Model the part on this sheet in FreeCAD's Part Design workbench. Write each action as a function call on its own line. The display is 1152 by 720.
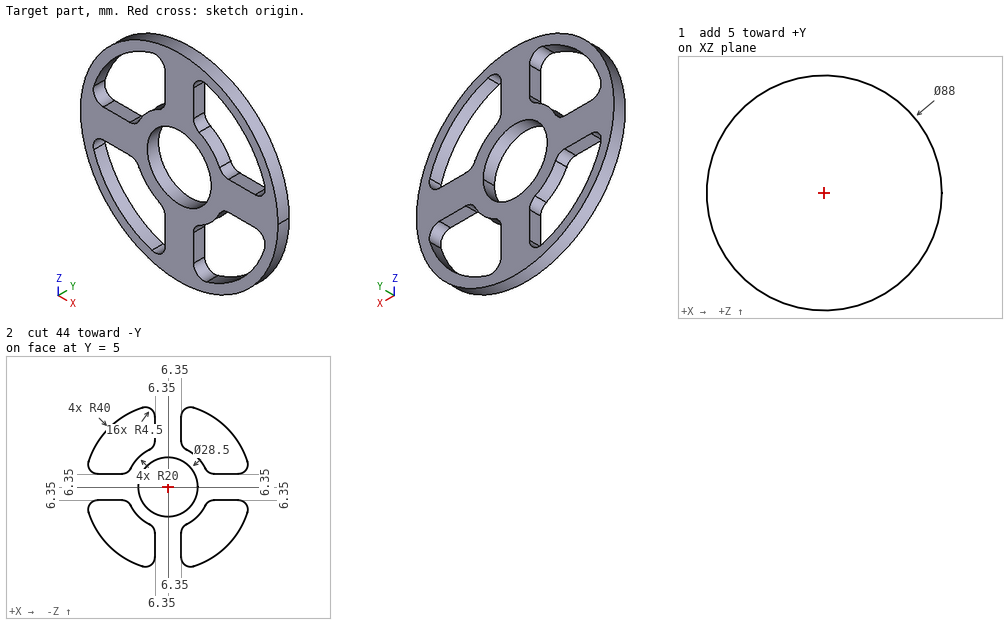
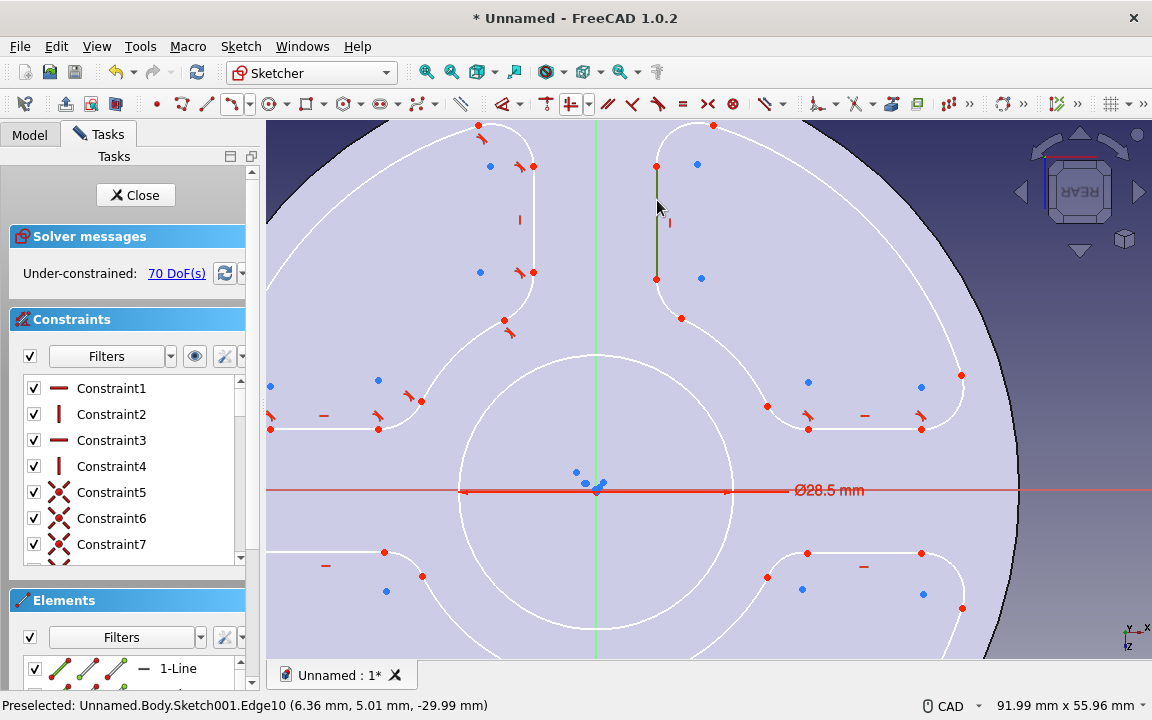
click(659, 150)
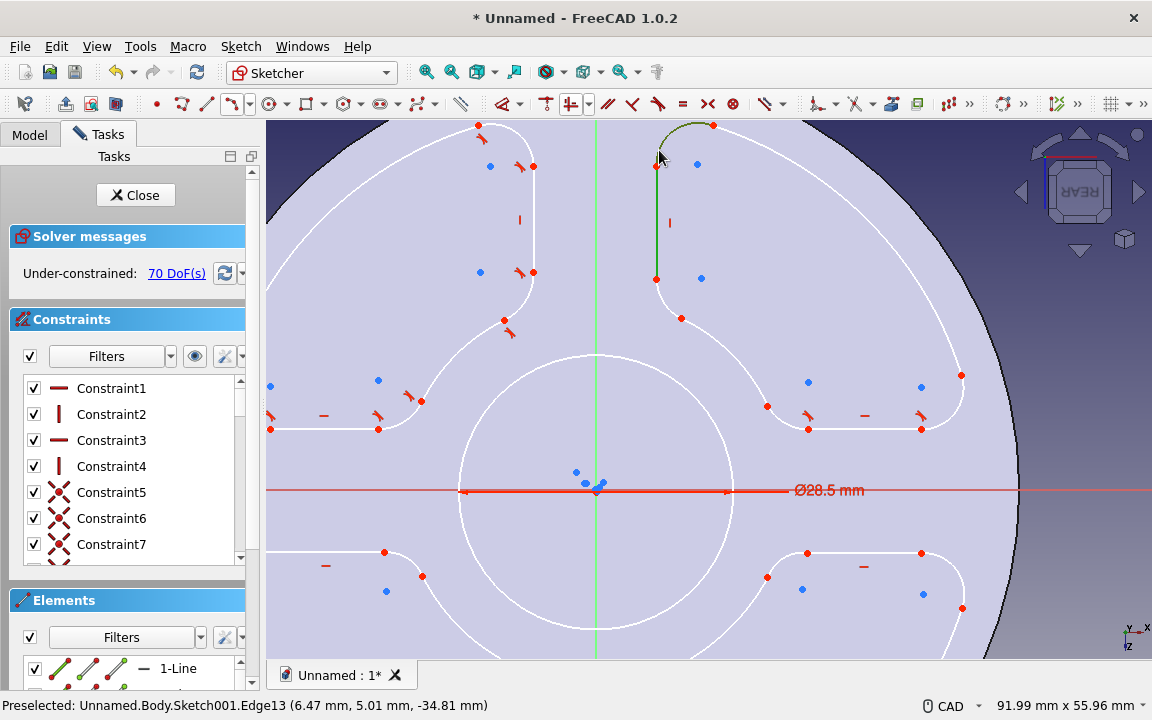
key(t)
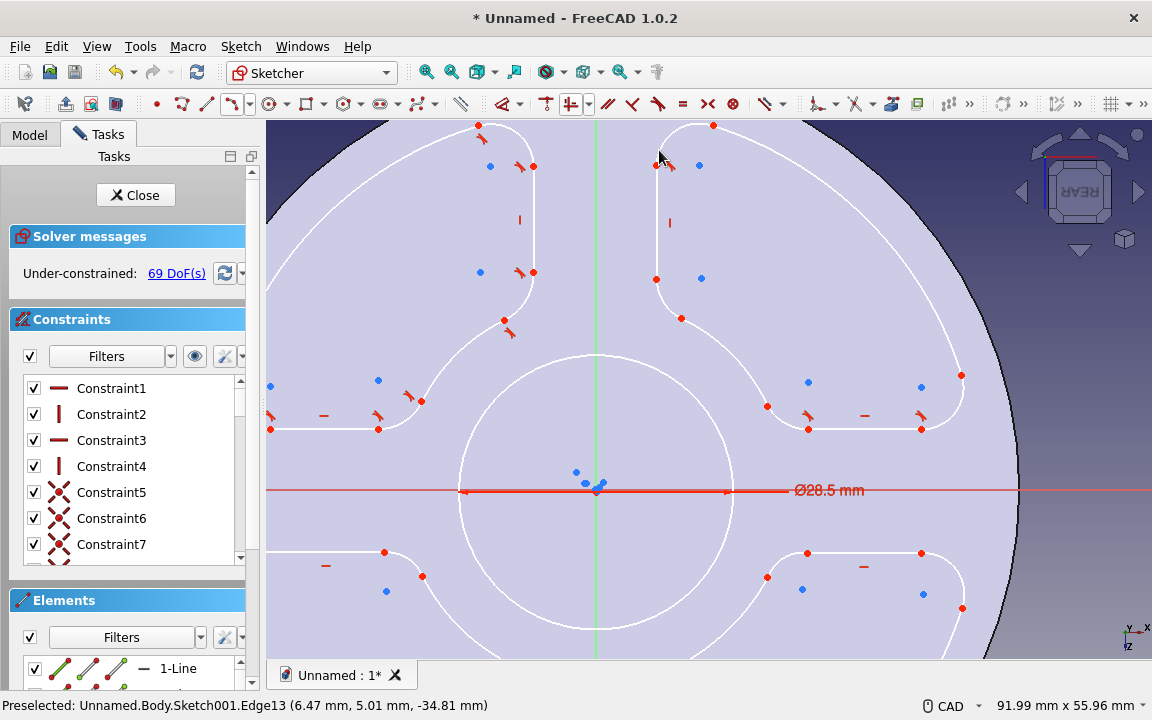
click(657, 200)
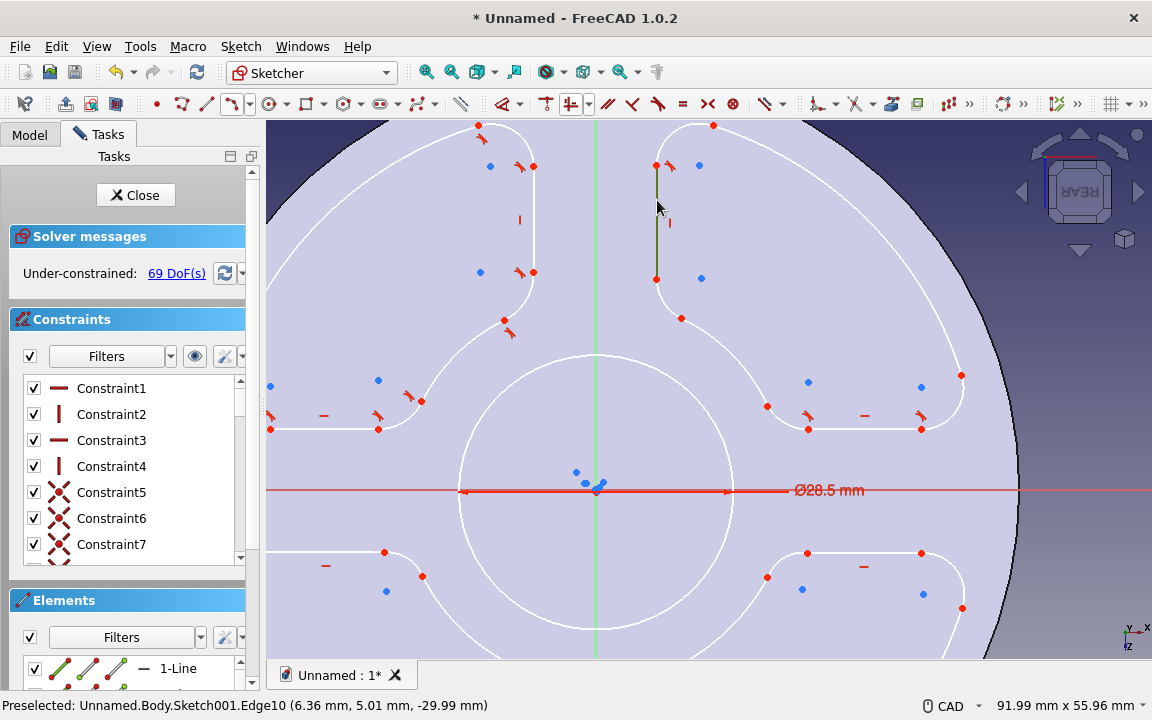
click(659, 294)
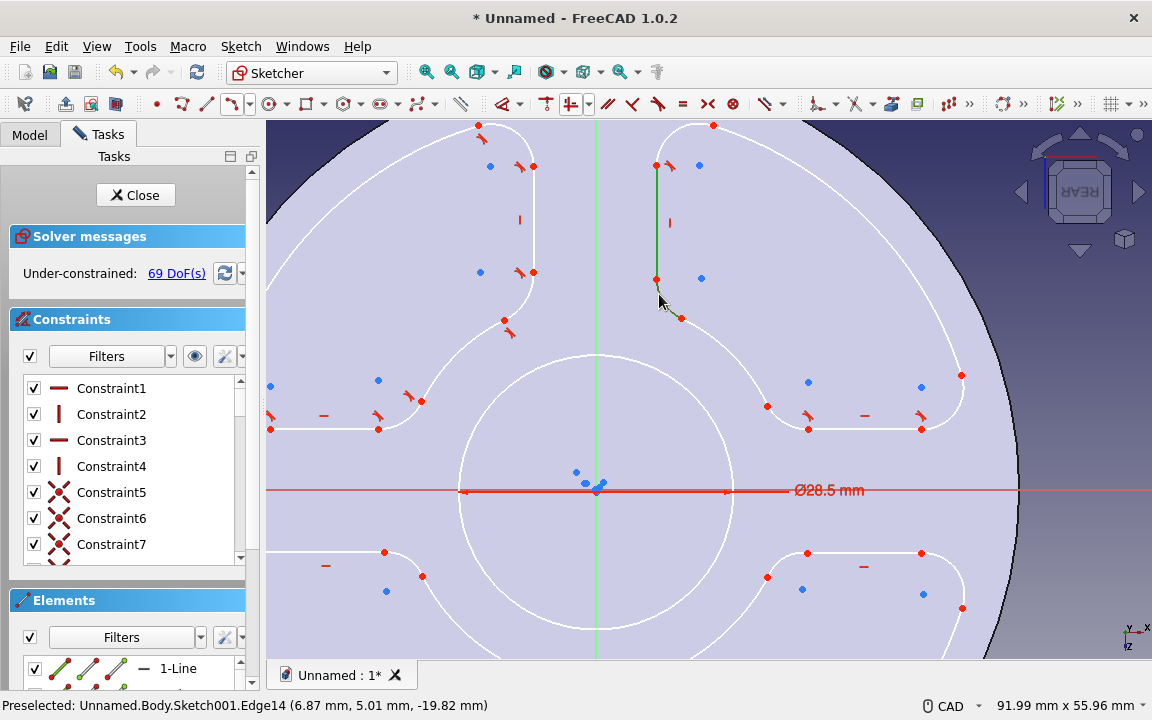
click(658, 104)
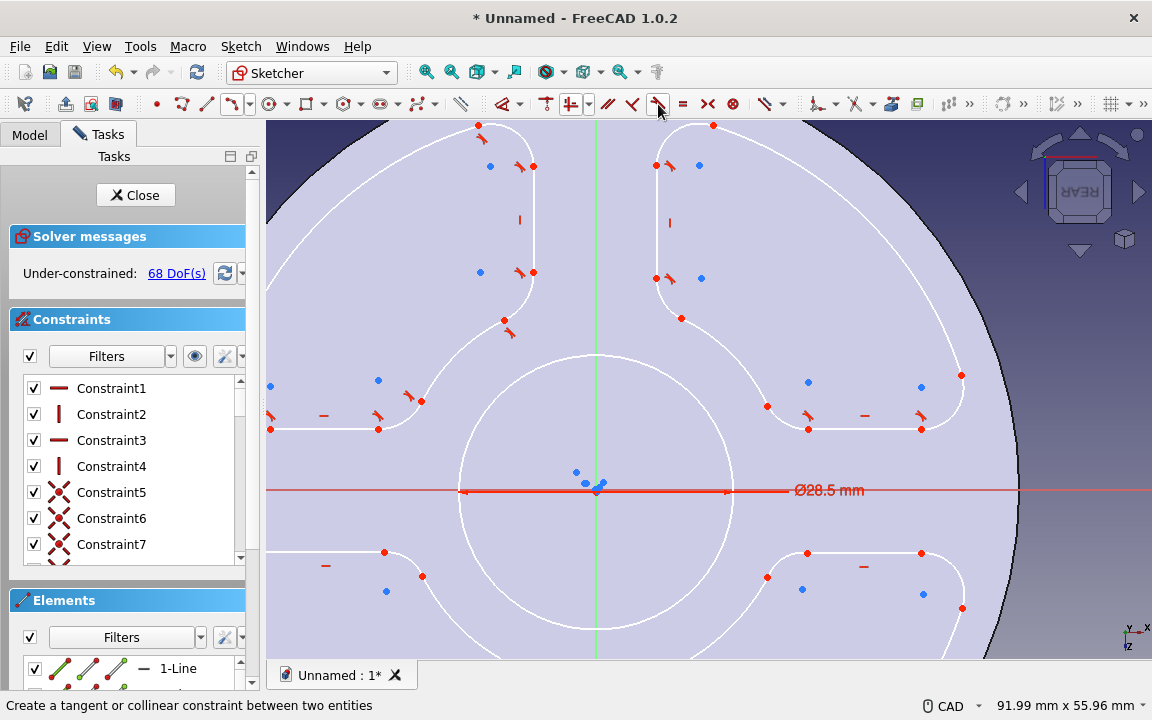
click(944, 423)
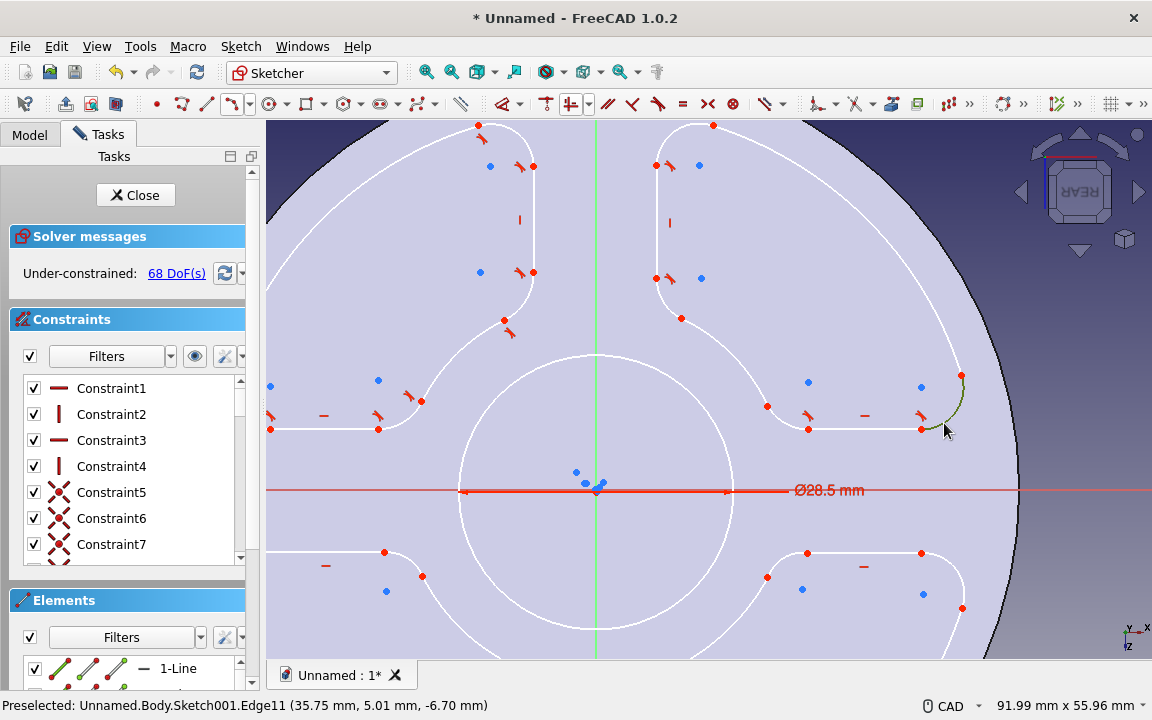
click(914, 277)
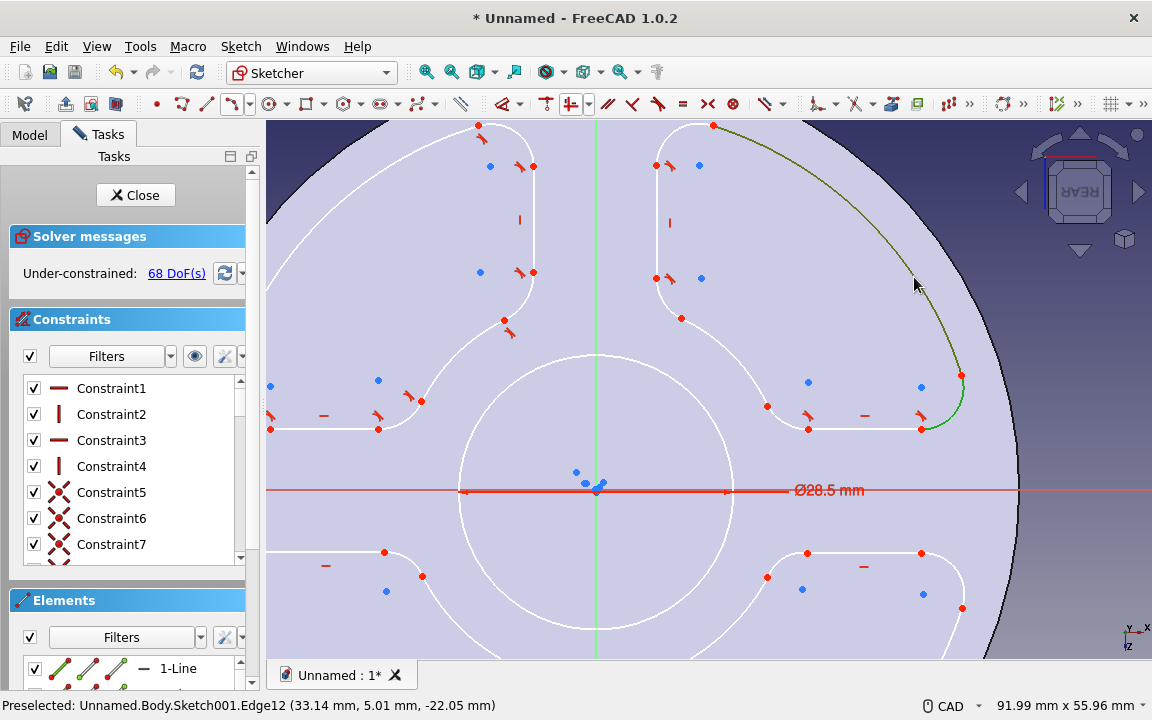
key(t)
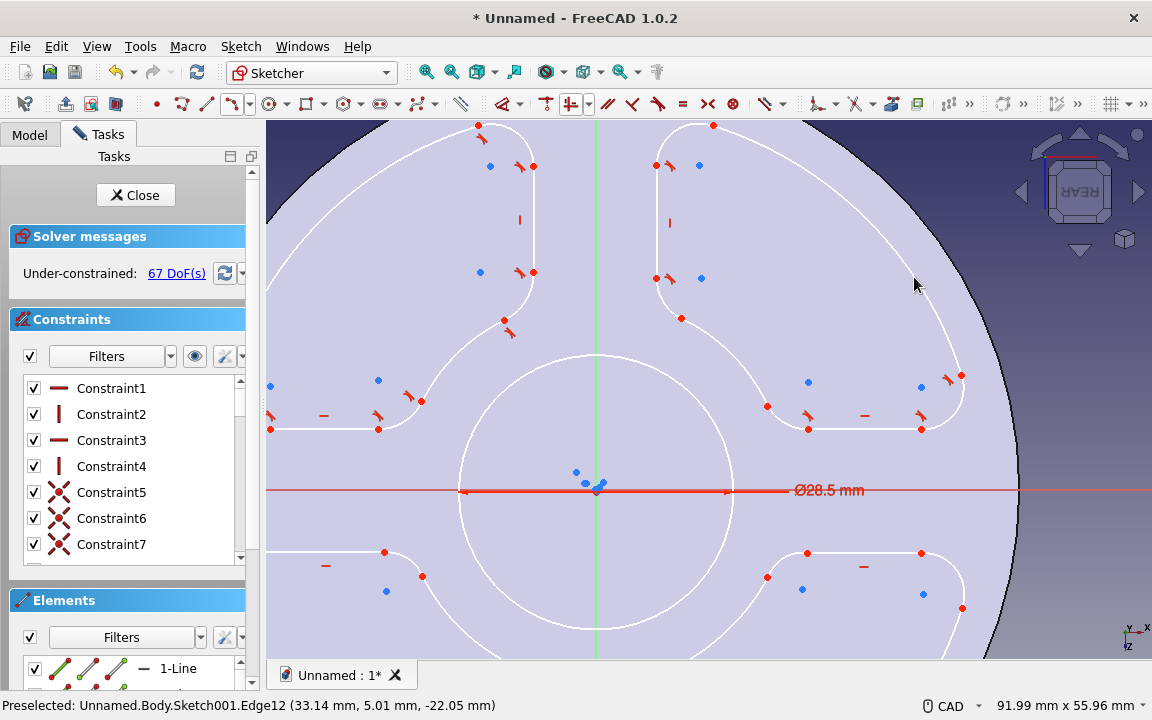
click(914, 277)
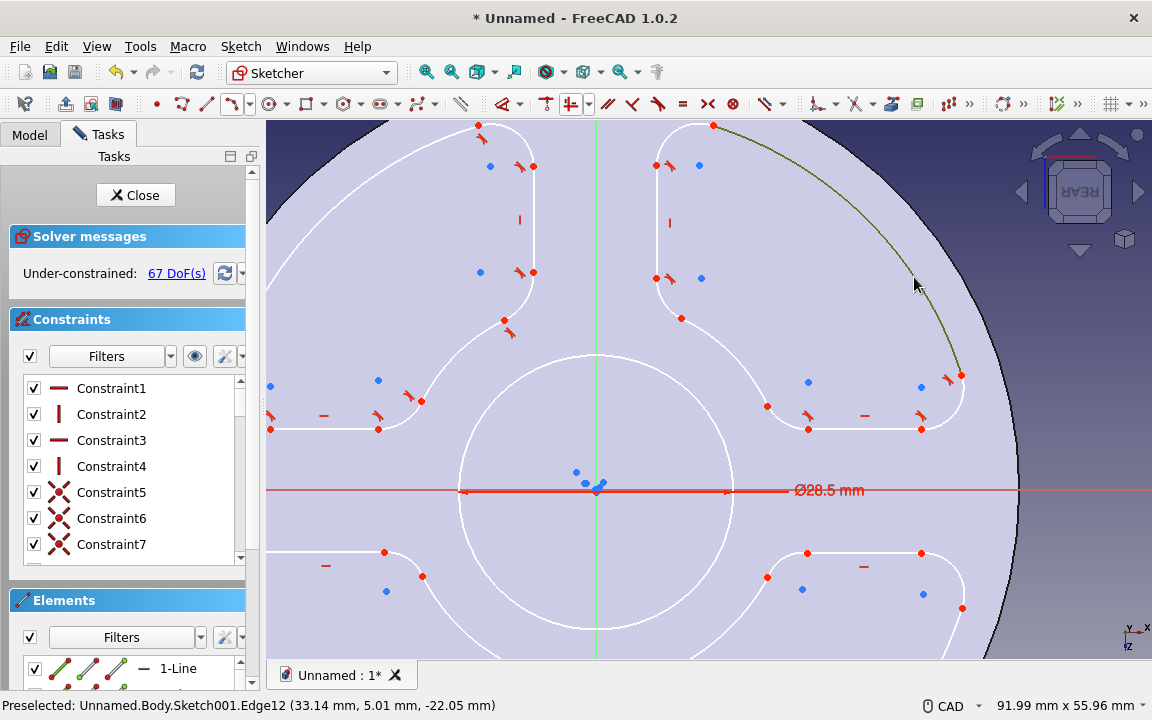
click(660, 150)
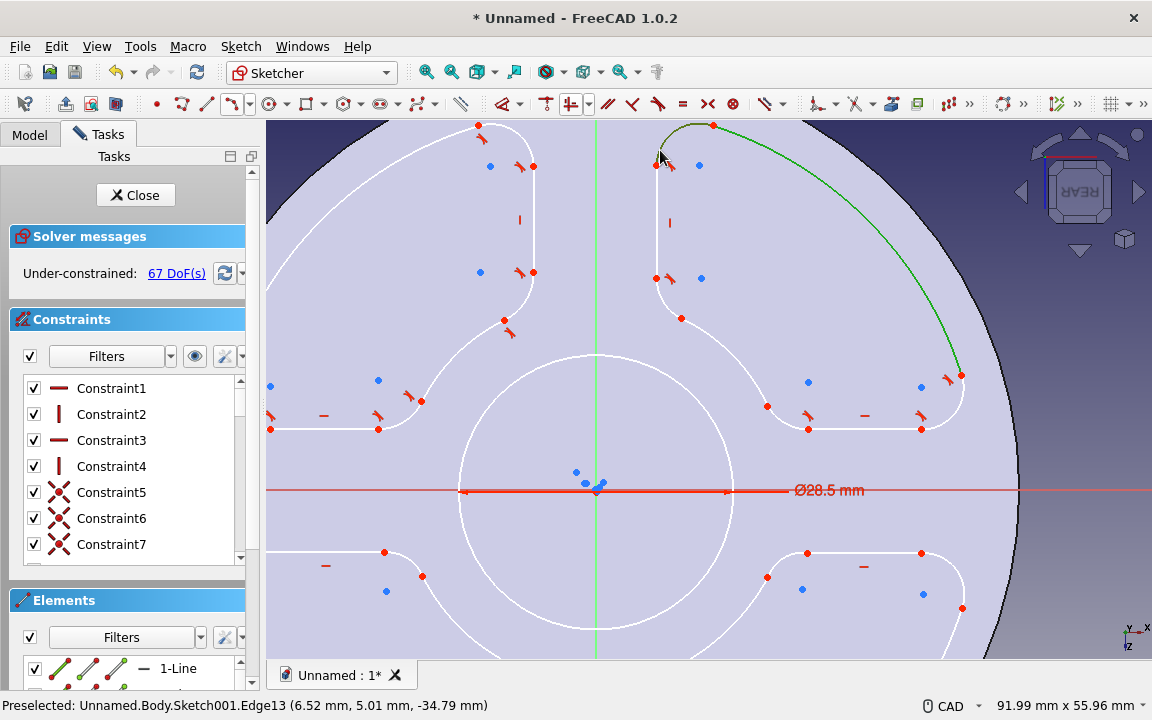
click(658, 104)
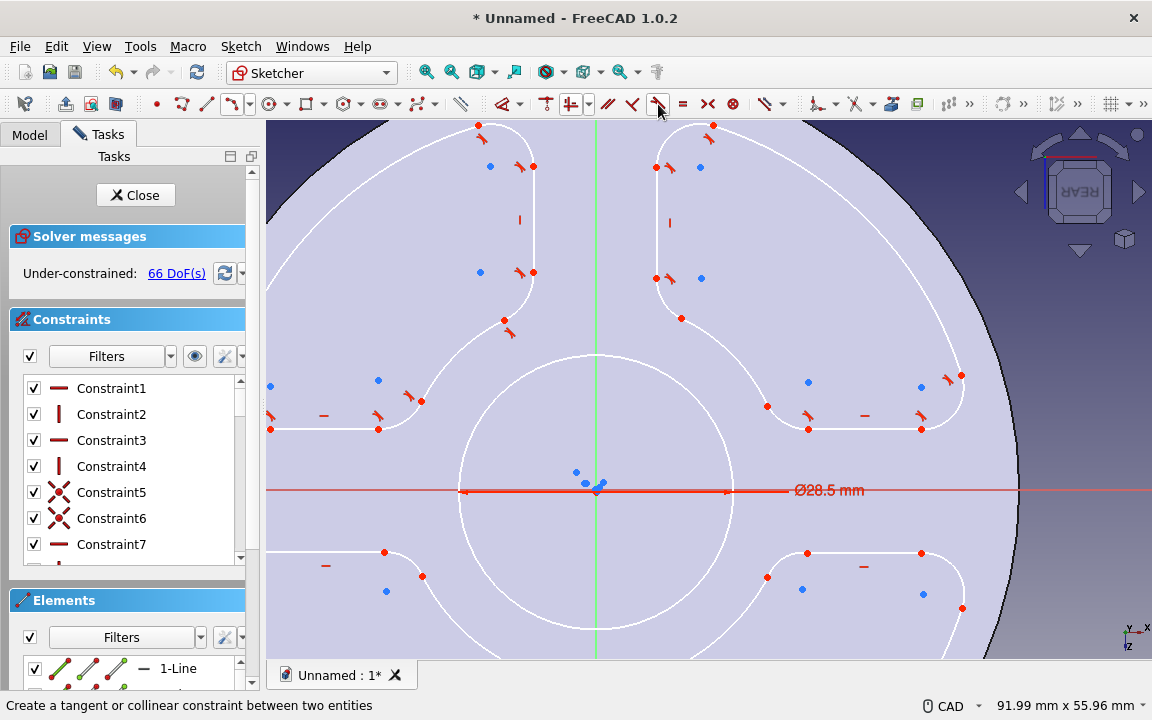
click(659, 293)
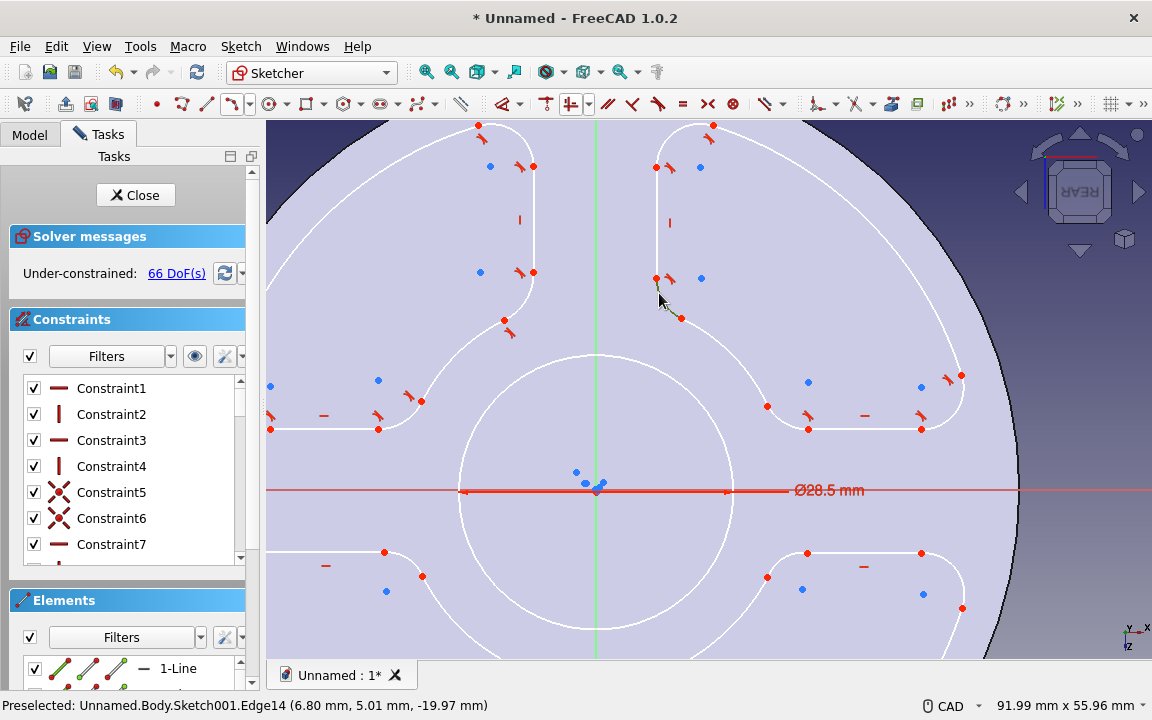
click(749, 374)